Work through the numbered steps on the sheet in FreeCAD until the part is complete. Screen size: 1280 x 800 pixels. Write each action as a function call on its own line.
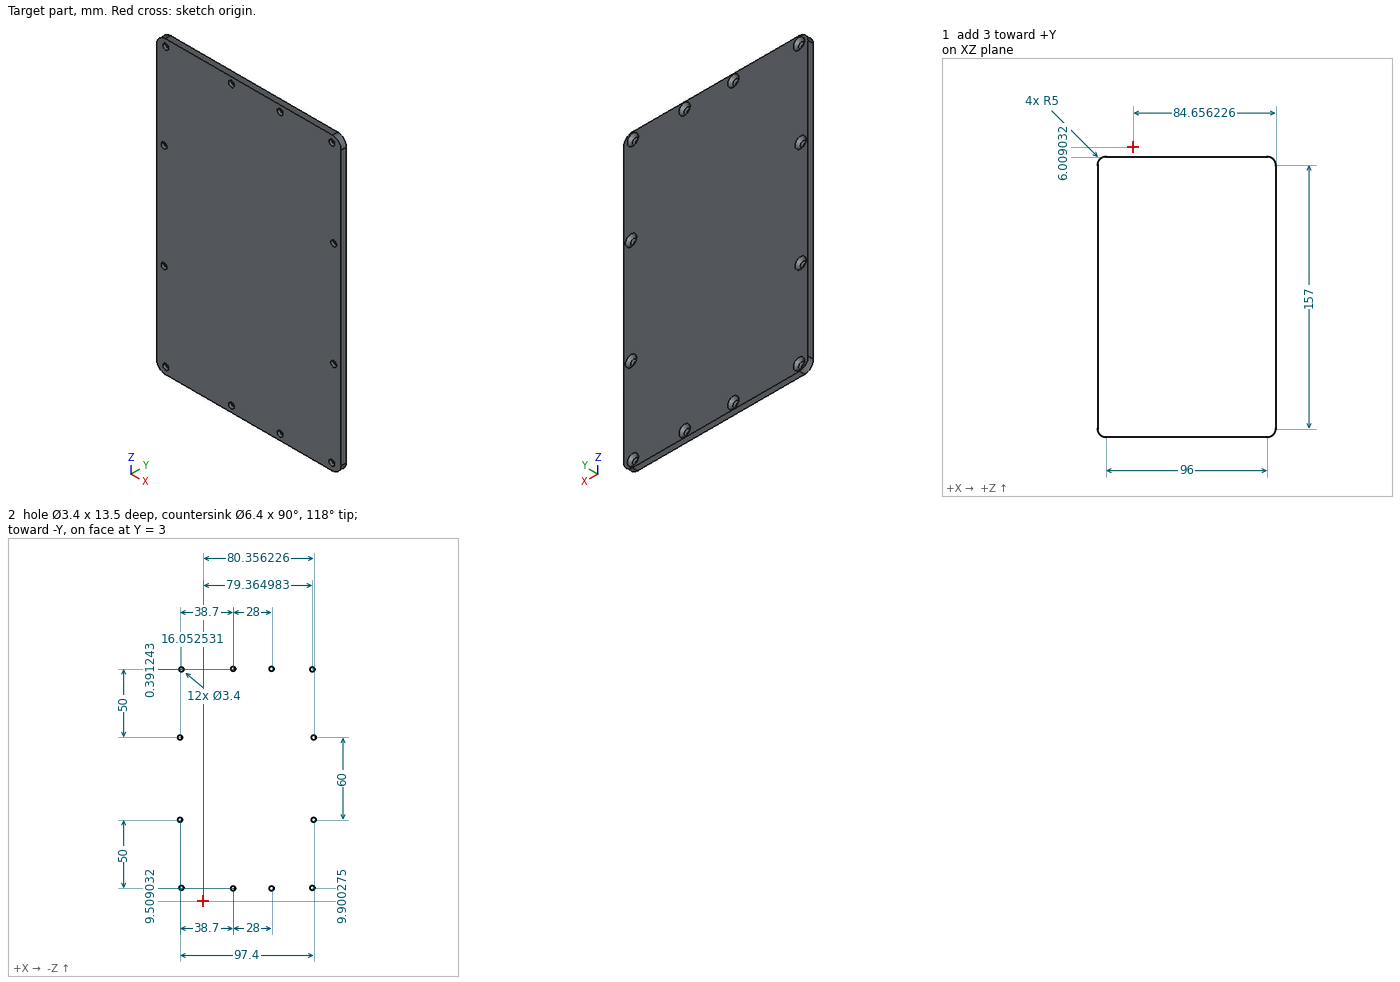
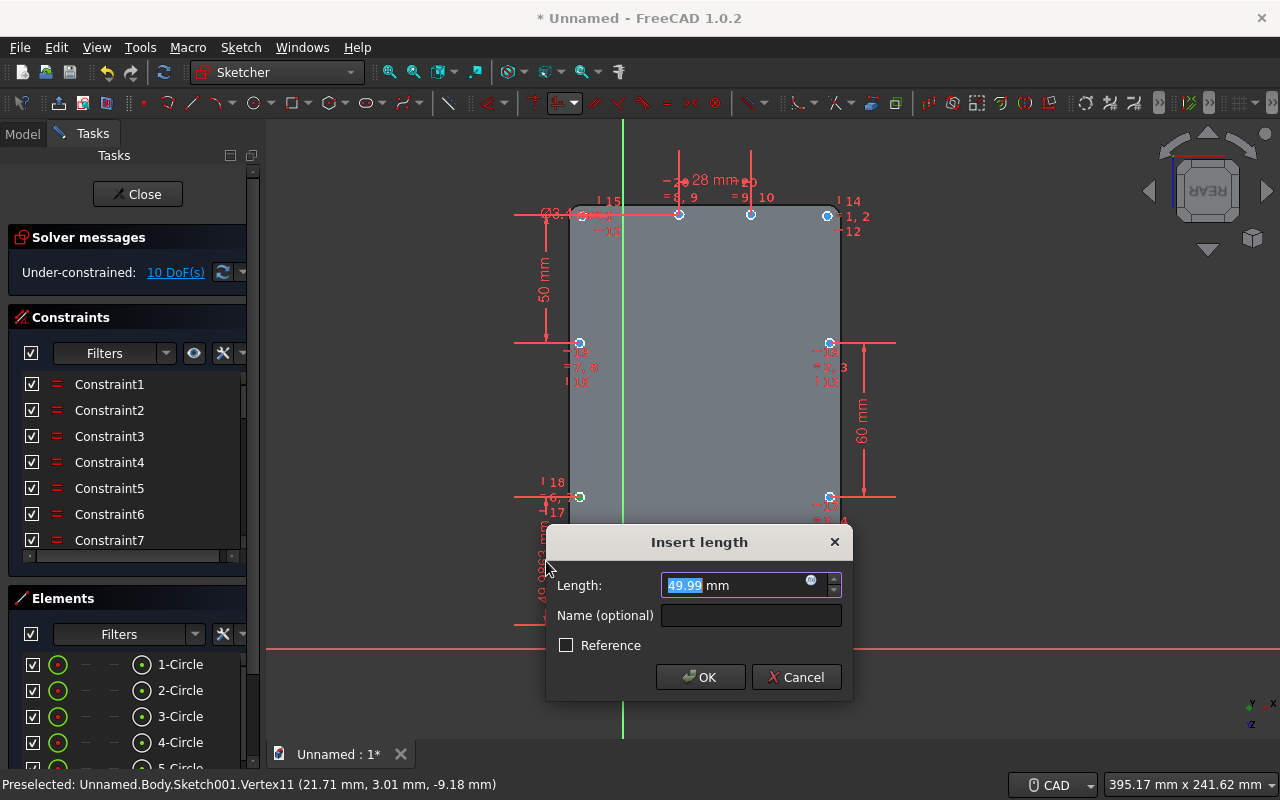
text(50)
key(Return)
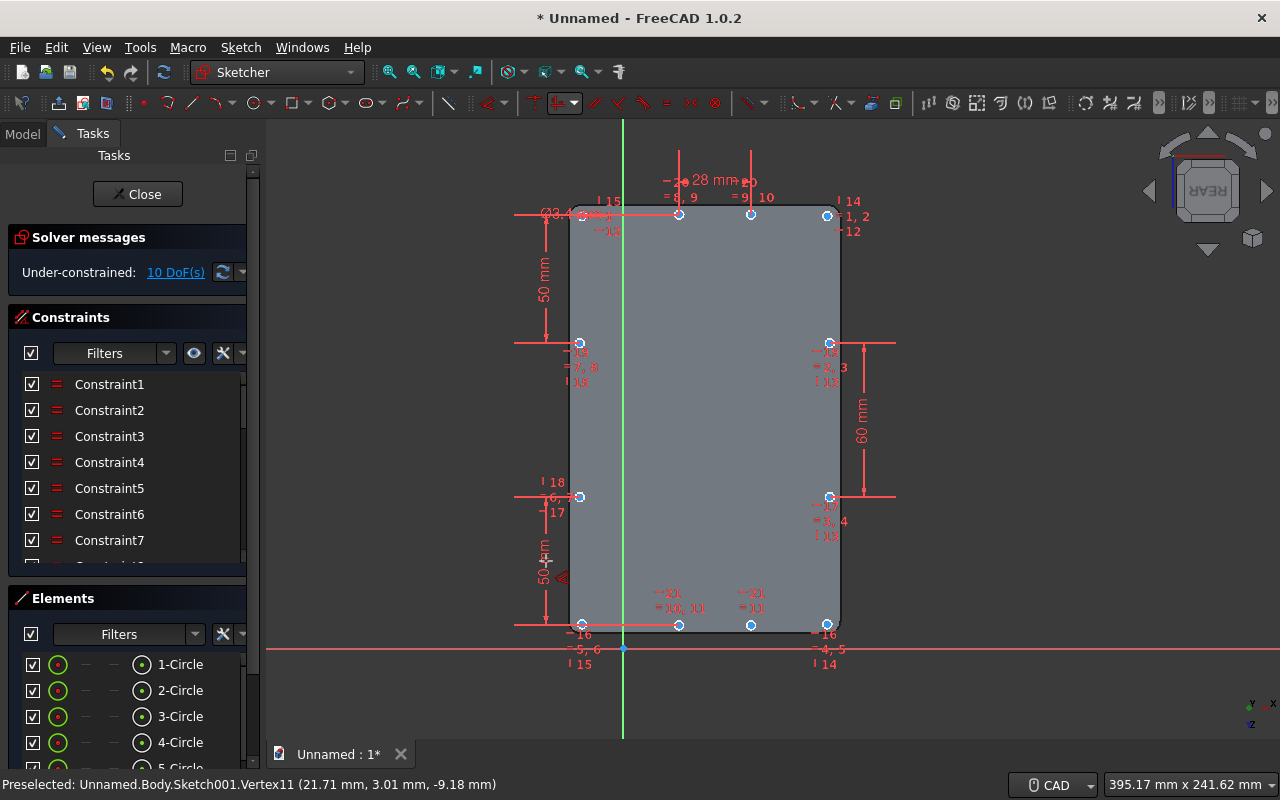
click(679, 625)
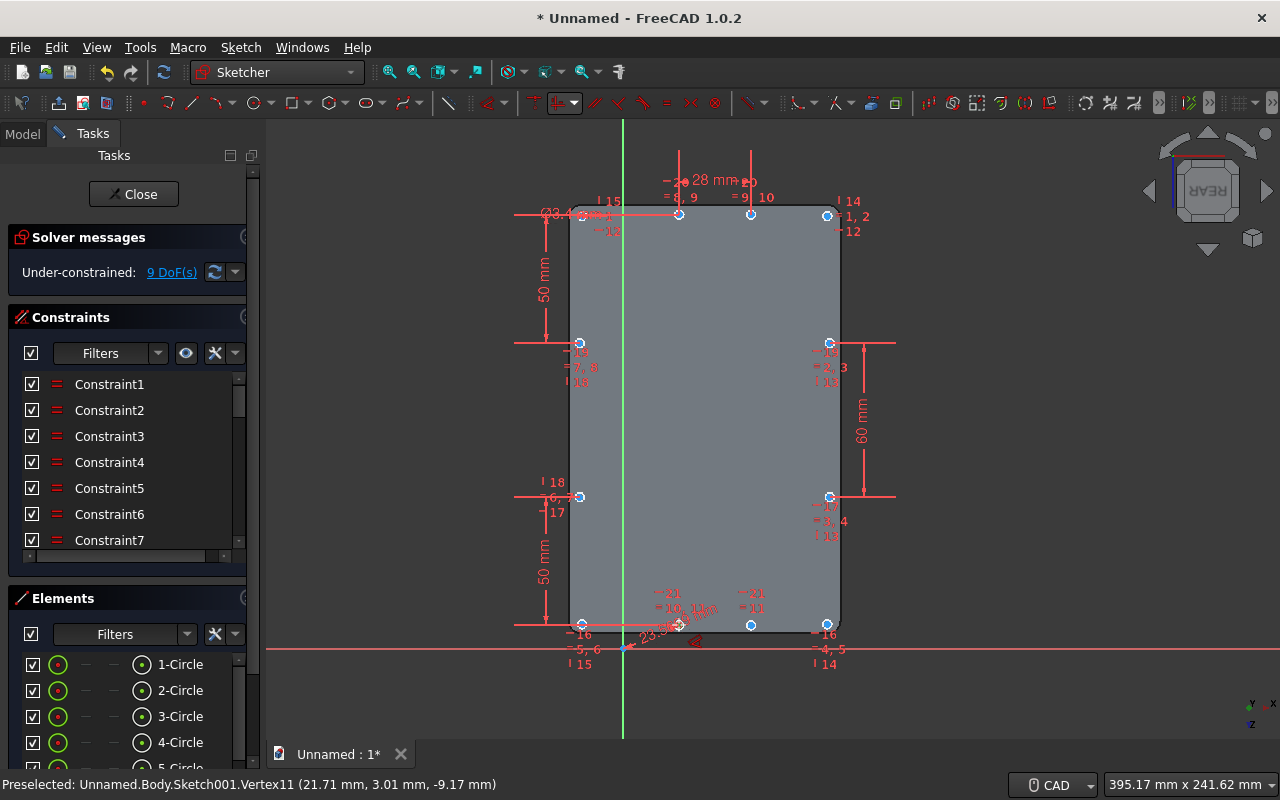
click(751, 625)
click(715, 591)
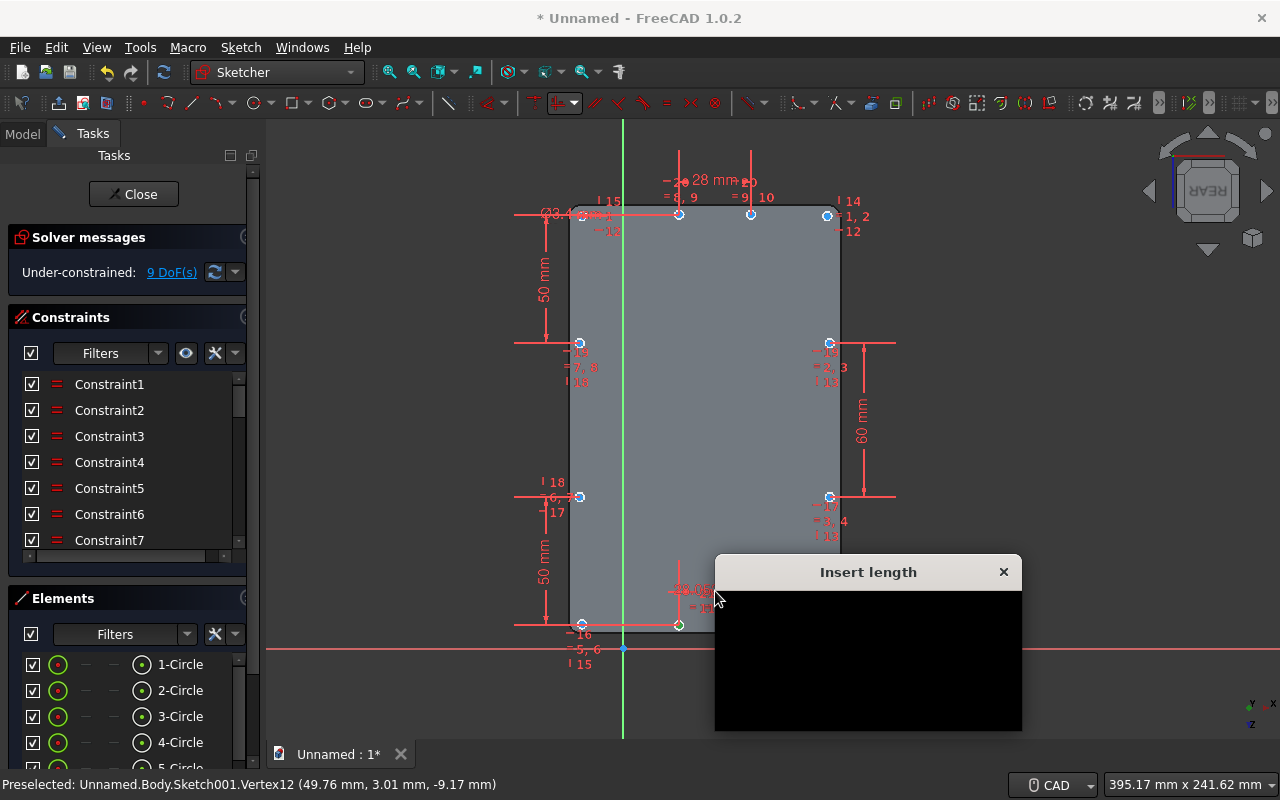
text(28)
key(Return)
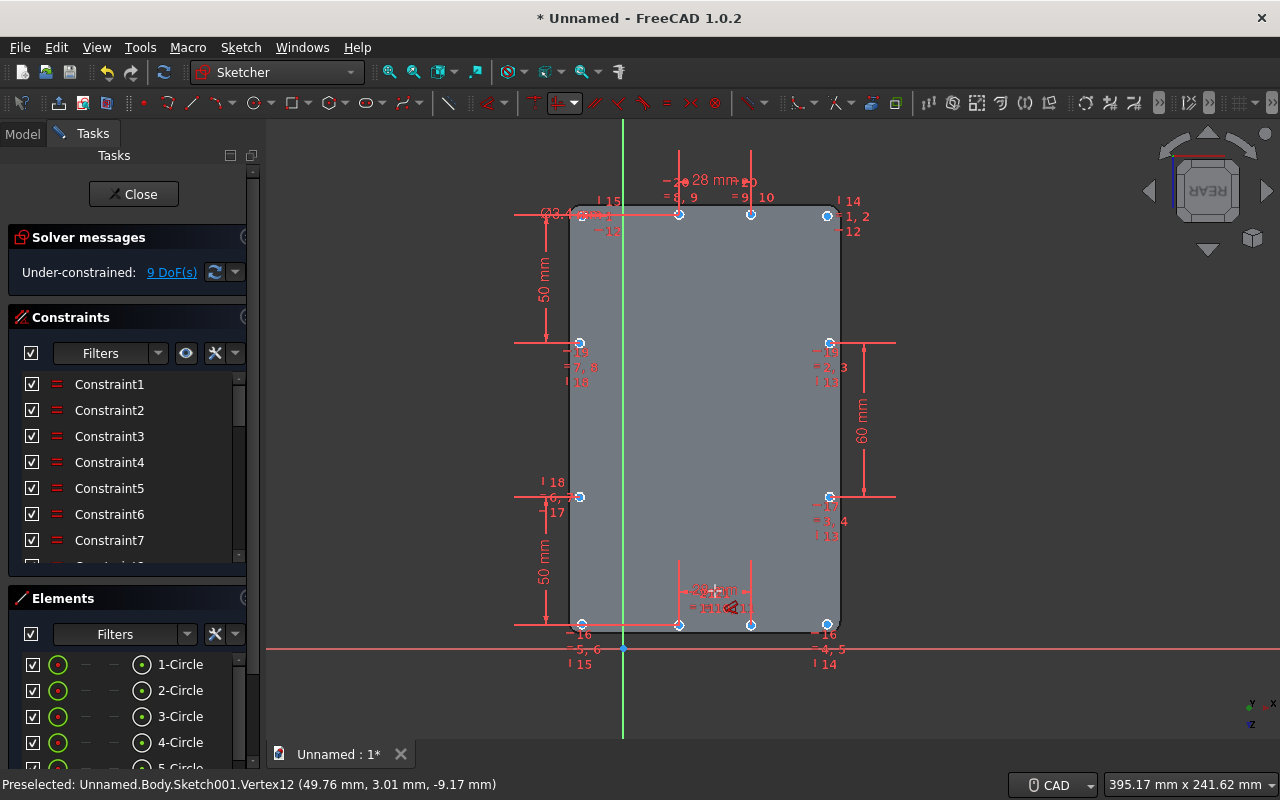
click(830, 497)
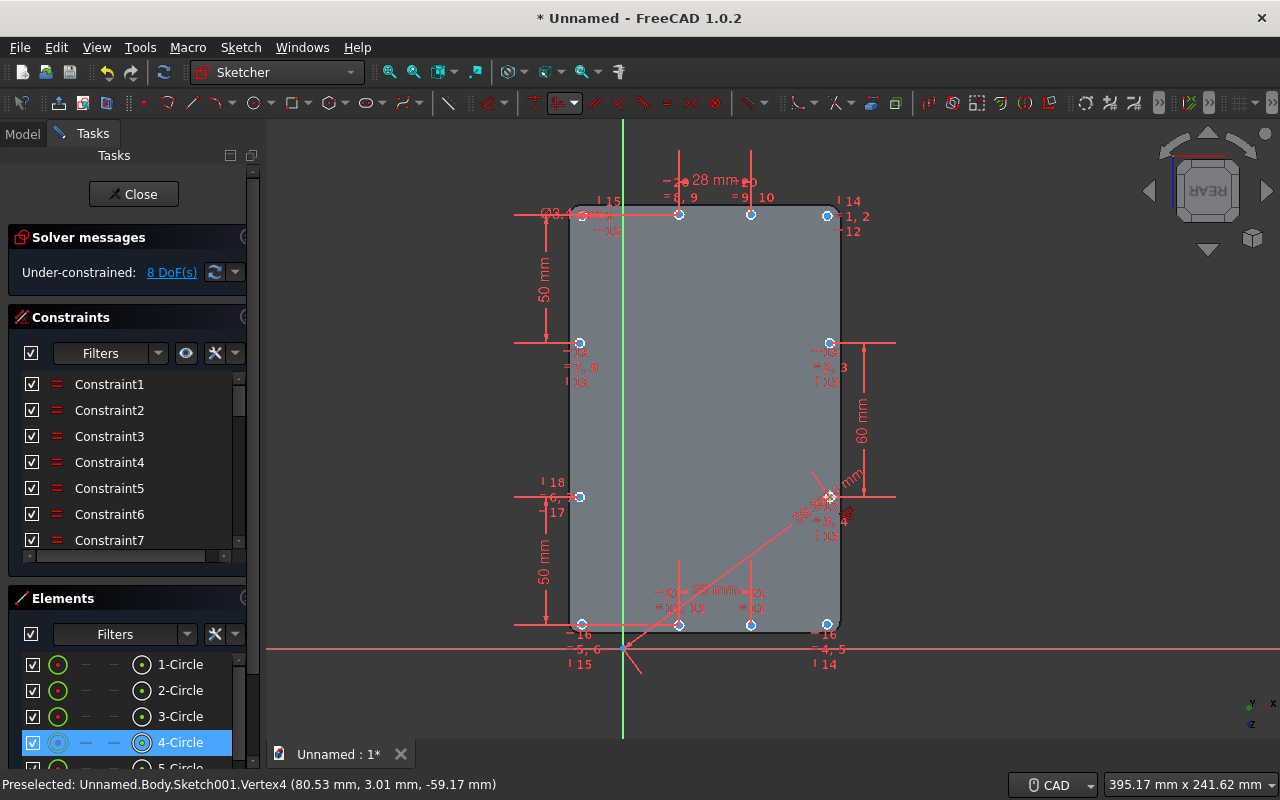
click(580, 497)
click(705, 531)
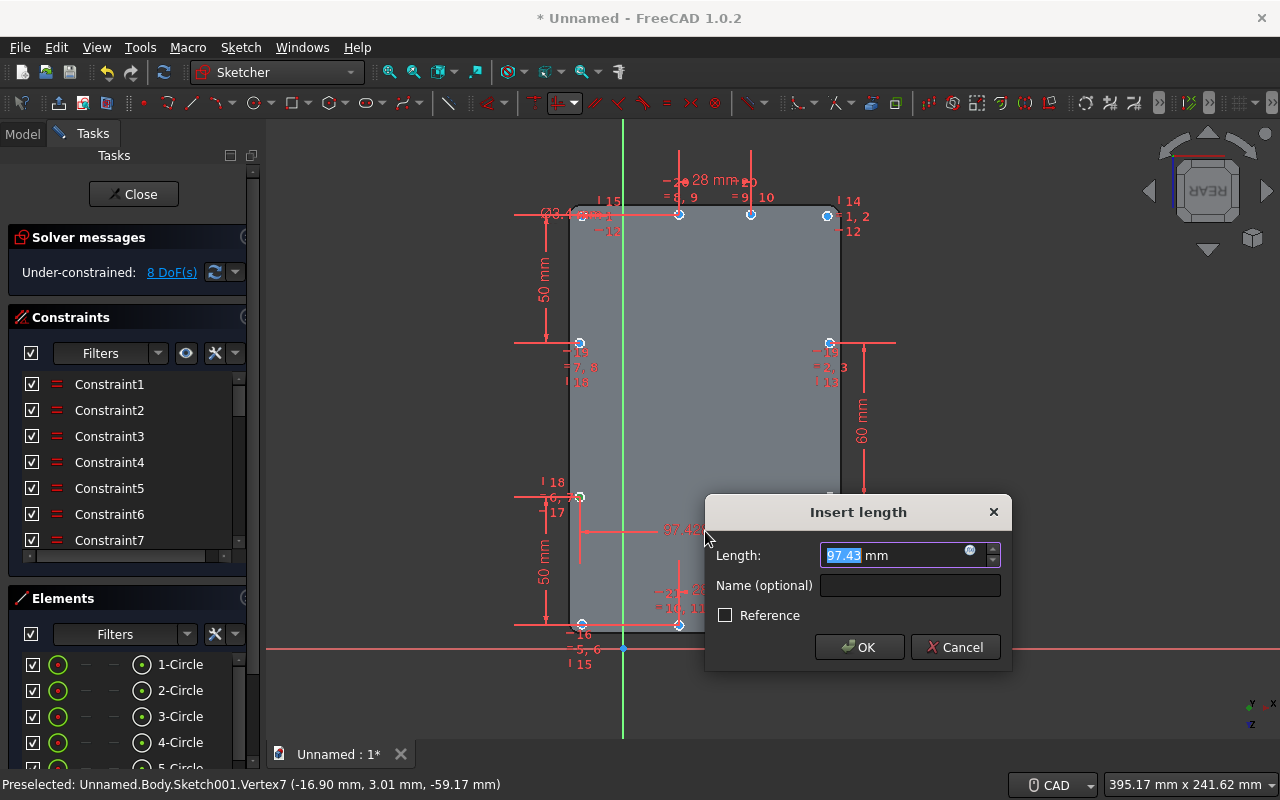
text(97.4)
key(Return)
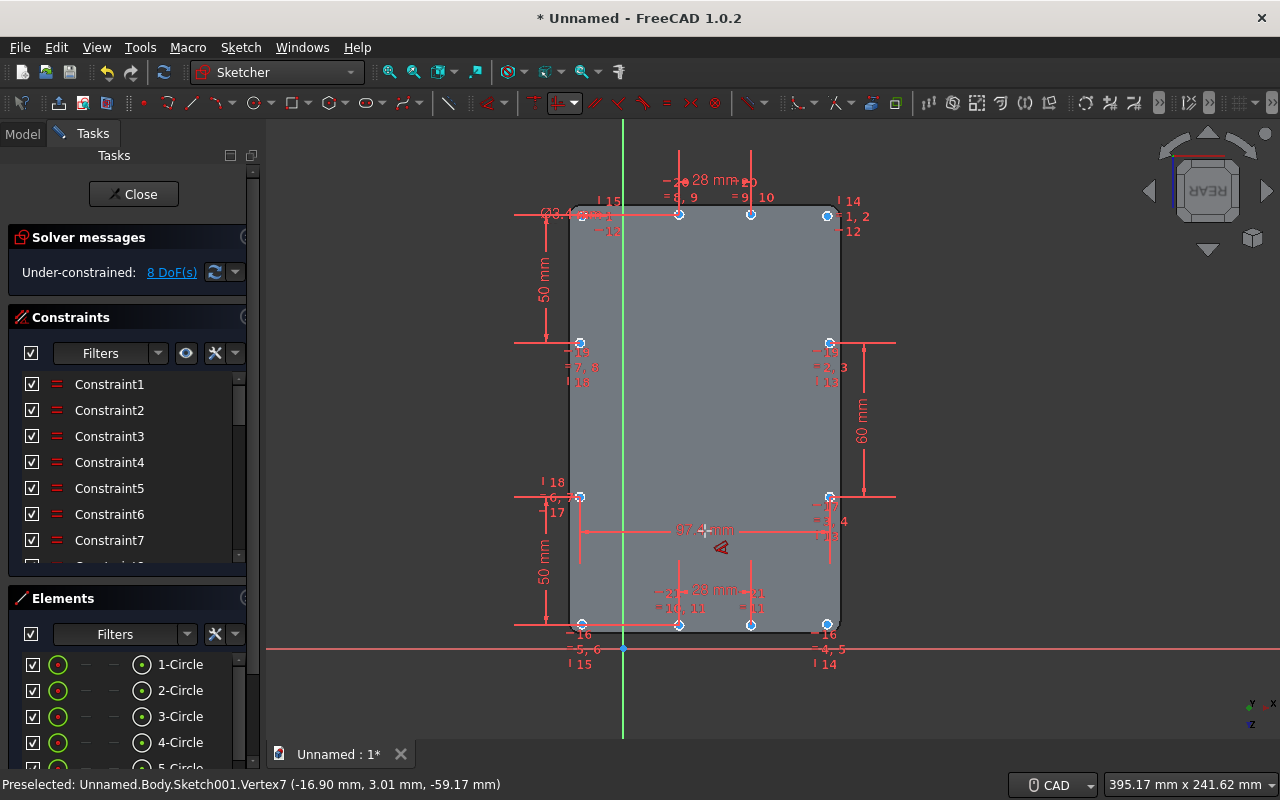
click(580, 343)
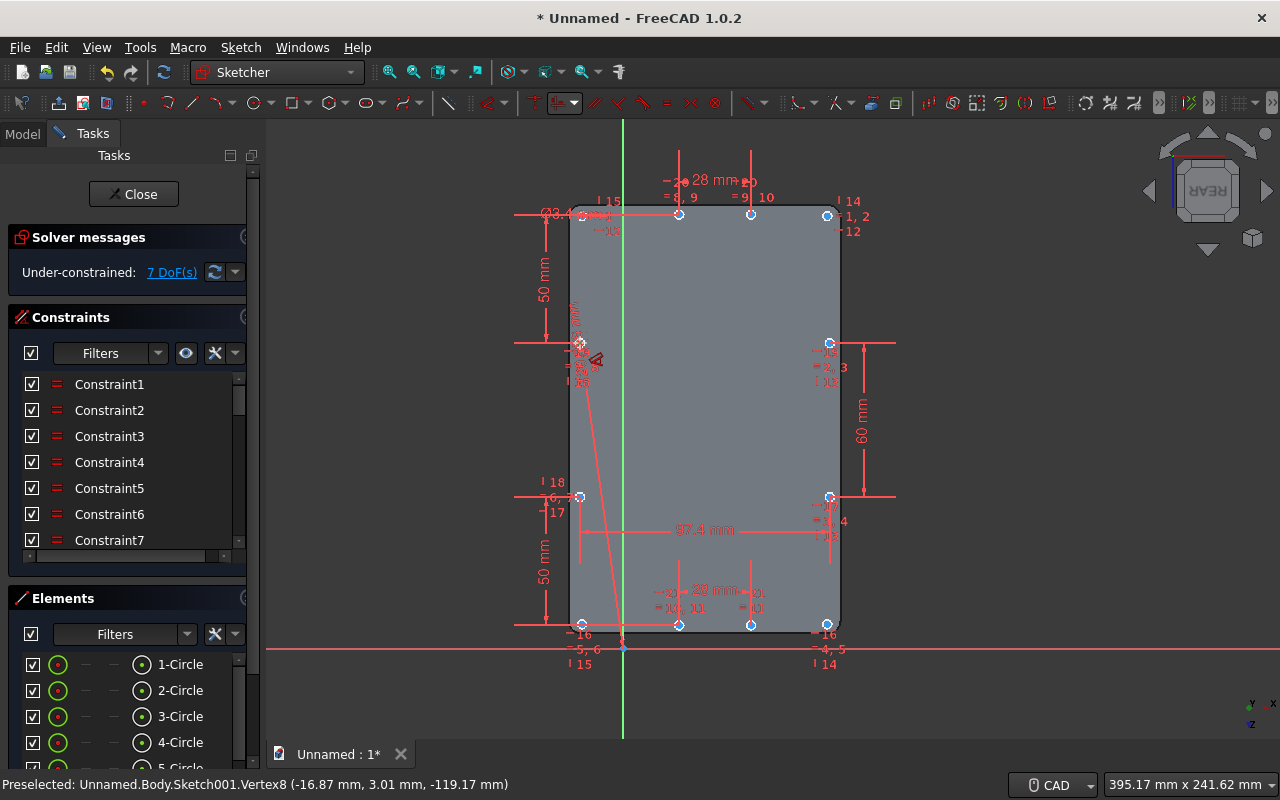
click(679, 215)
click(607, 181)